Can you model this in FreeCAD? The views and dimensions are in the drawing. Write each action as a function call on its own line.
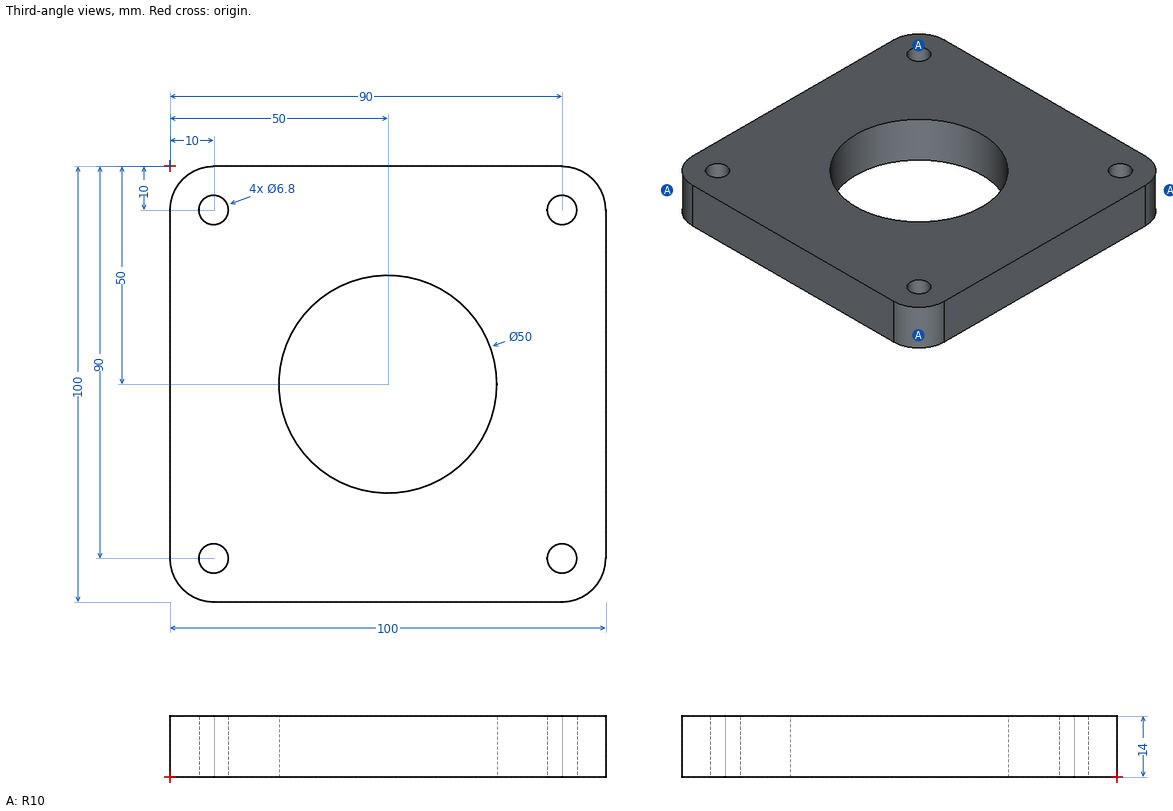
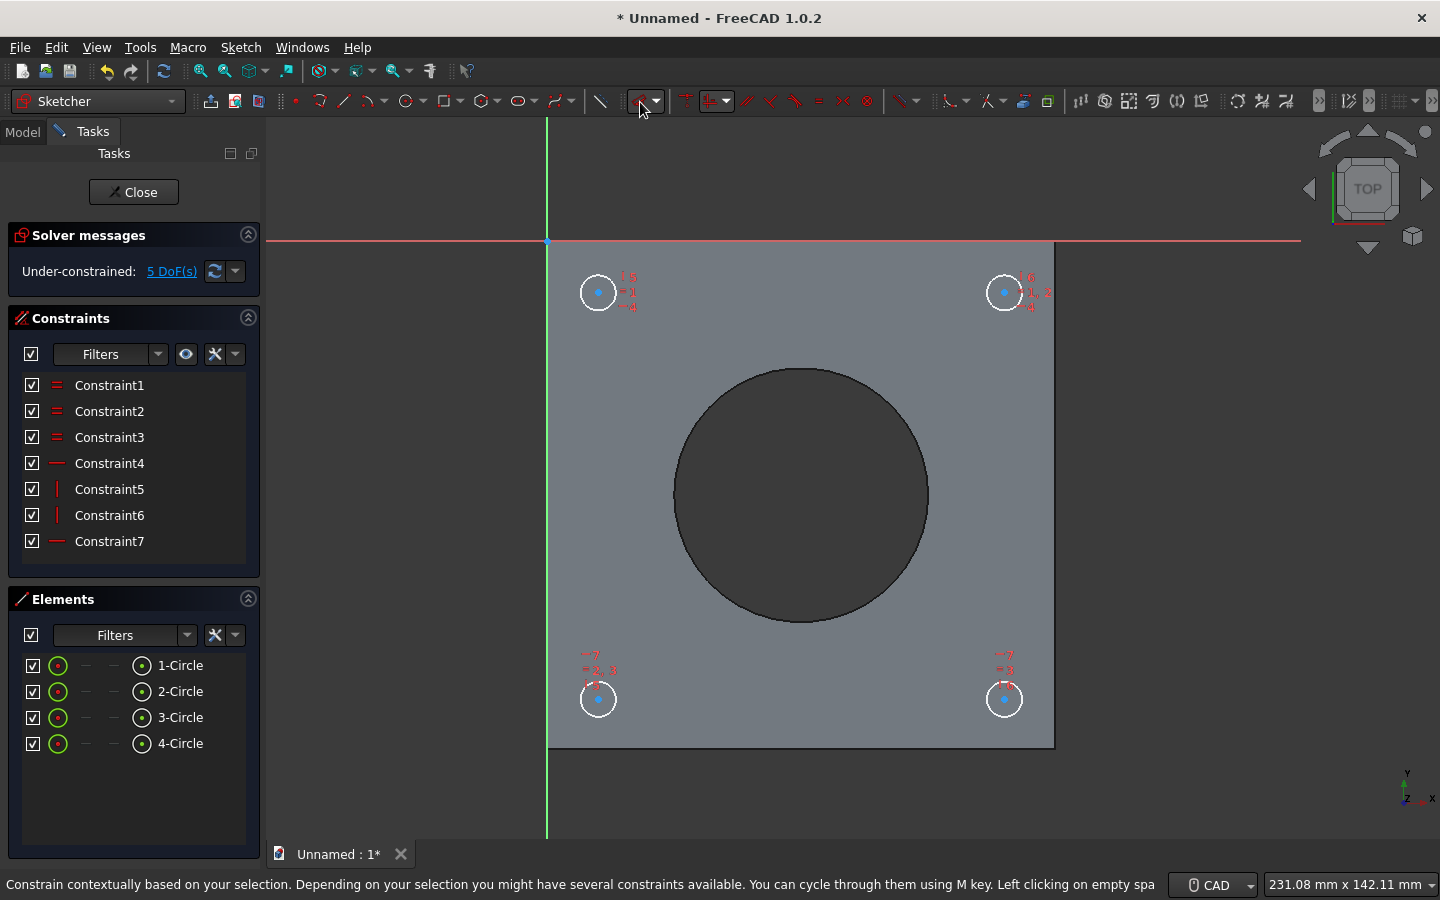
click(611, 280)
click(633, 257)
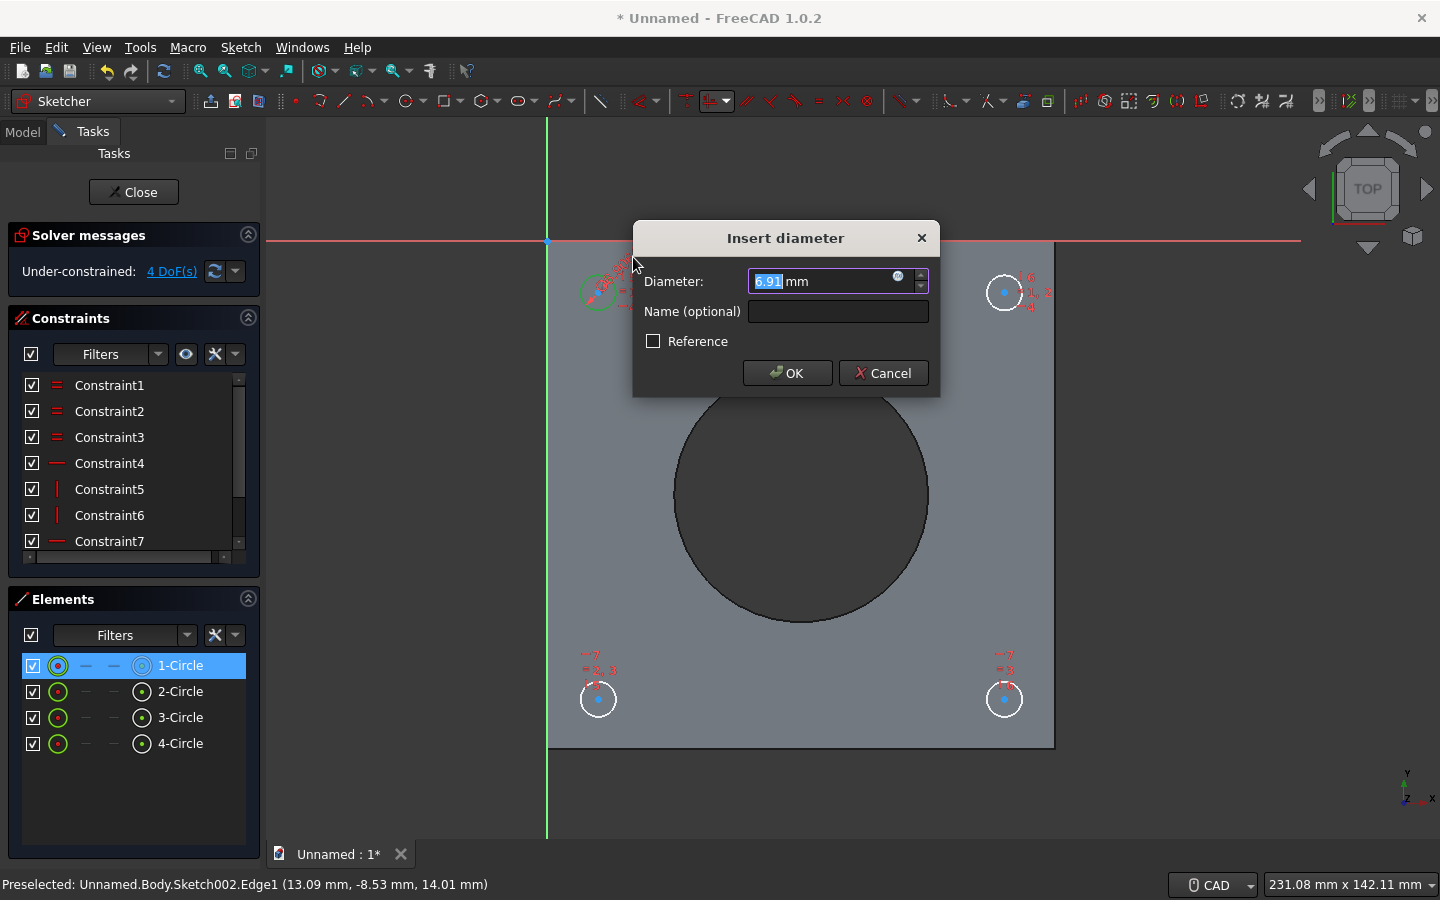
text(6.8)
key(Return)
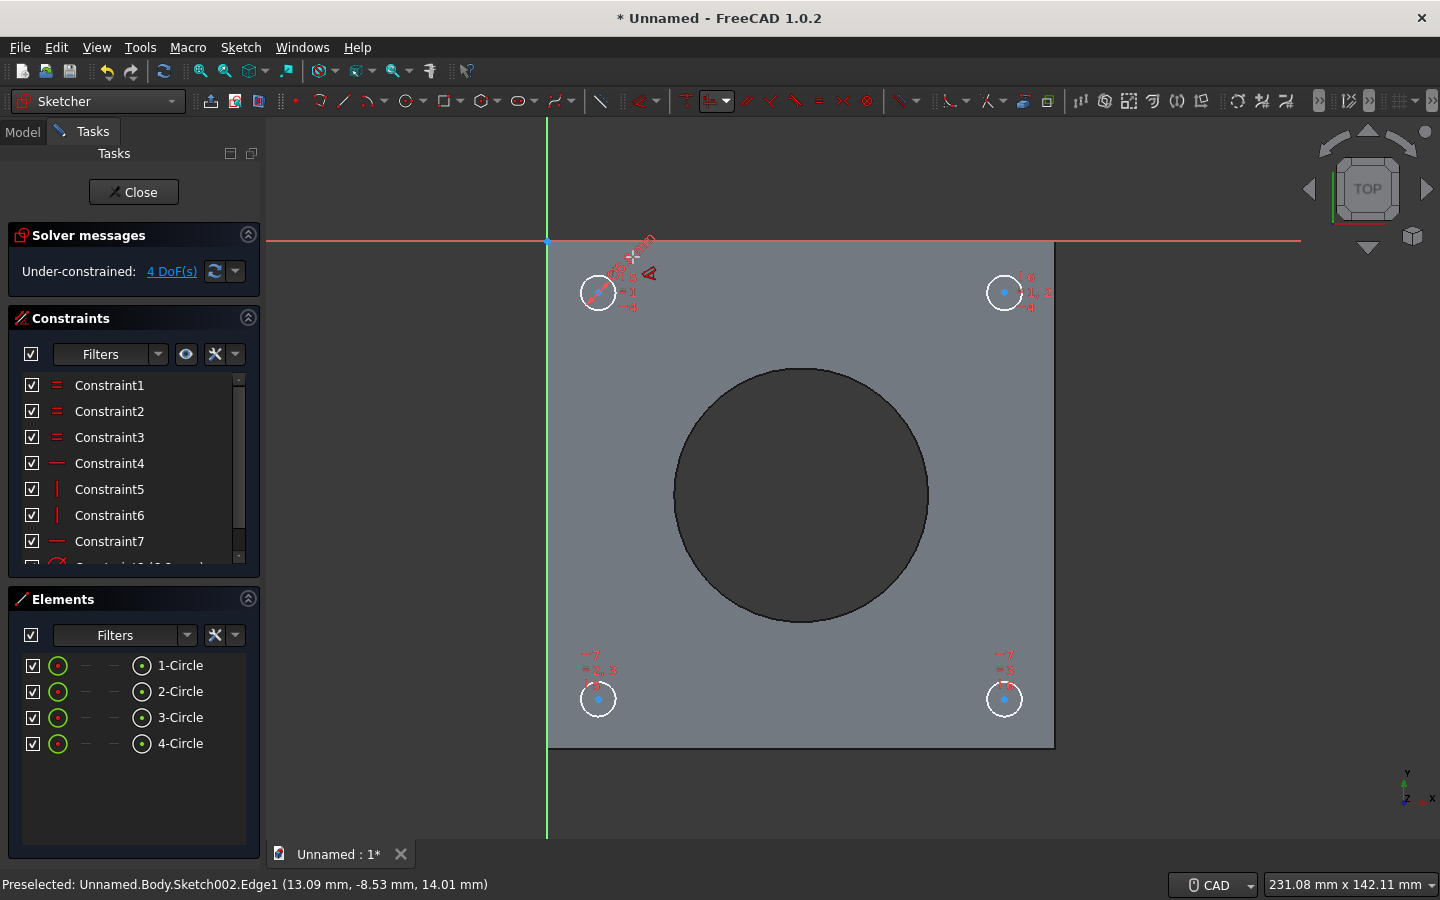
click(598, 293)
click(573, 207)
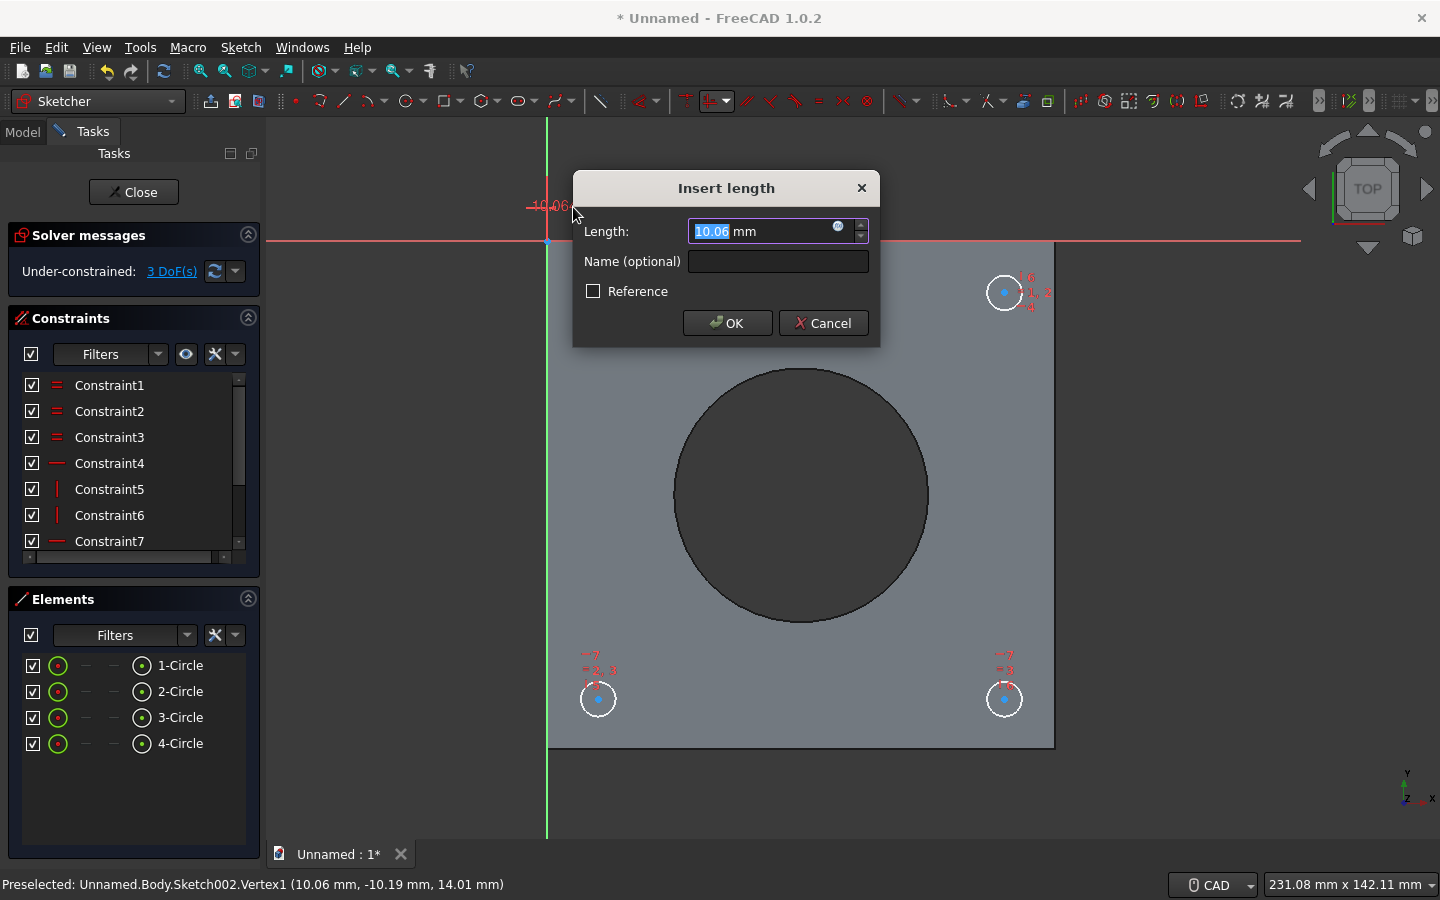
text(10)
key(Return)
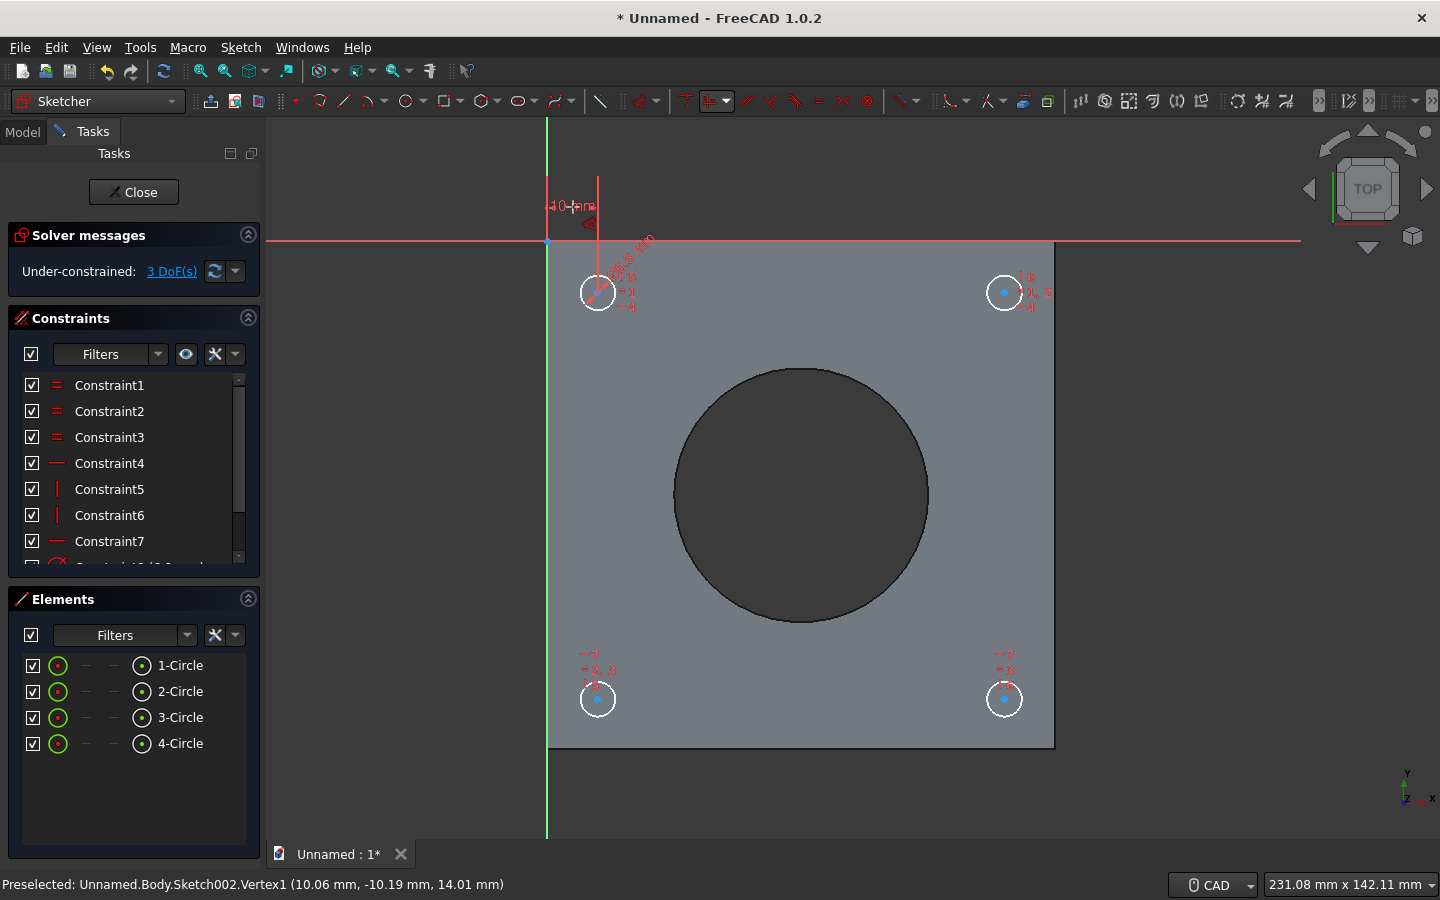
click(598, 293)
click(513, 267)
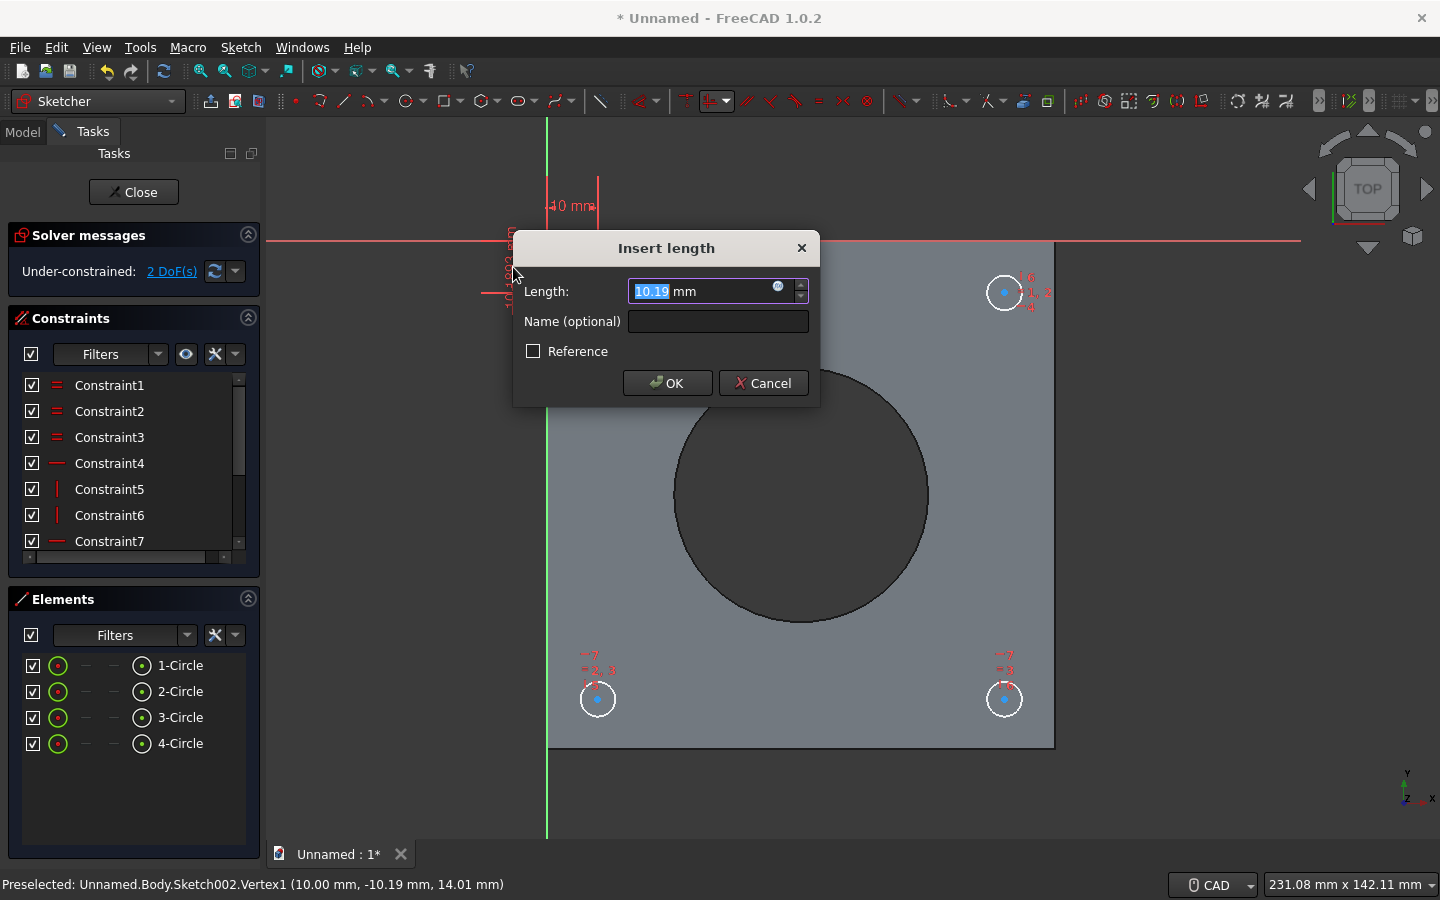
text(10)
key(Return)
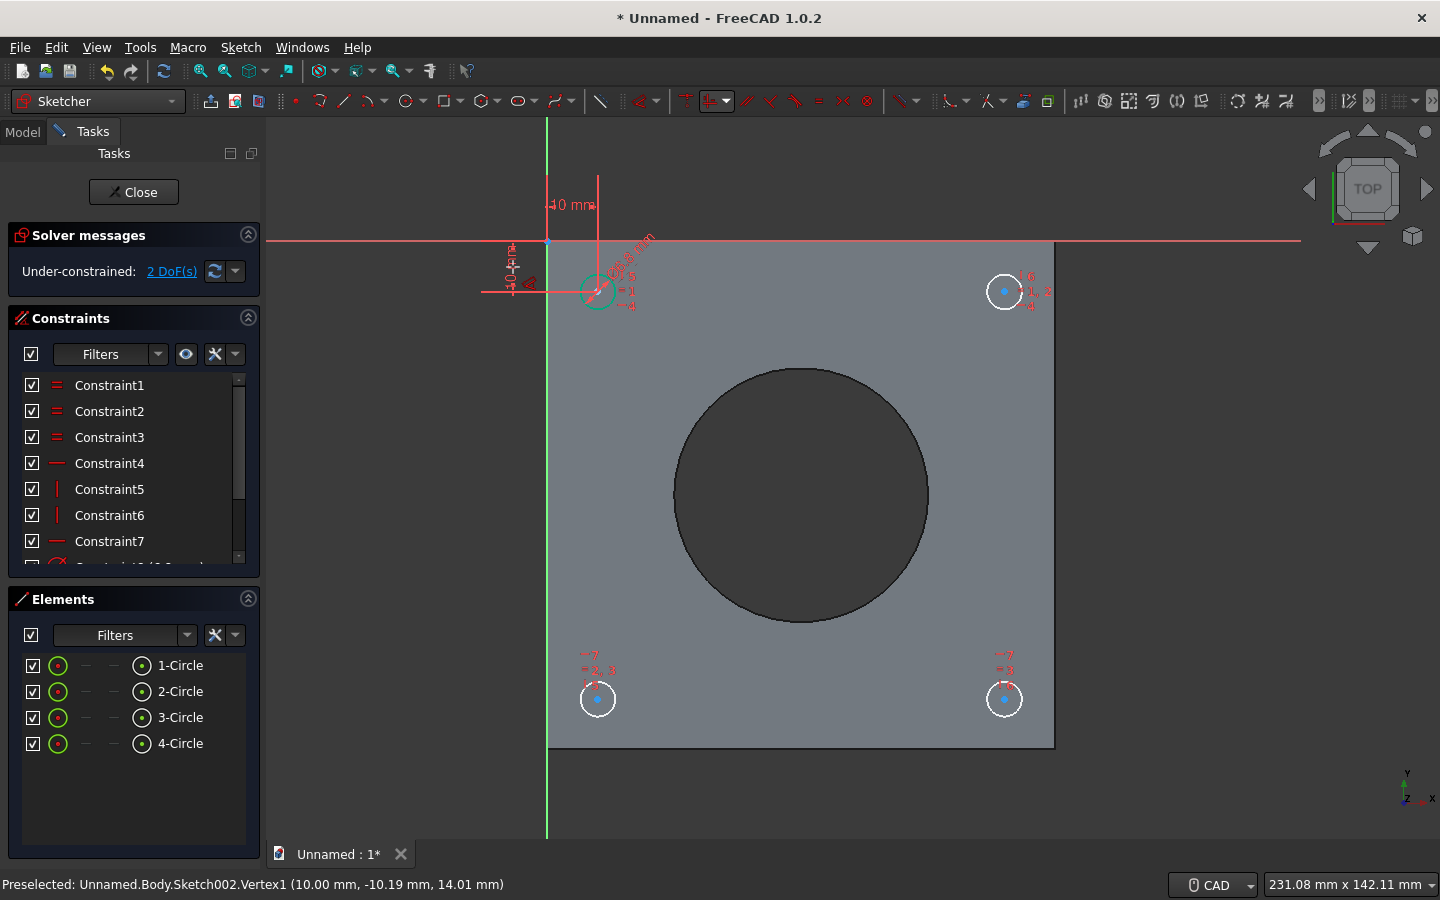
click(1005, 292)
click(776, 207)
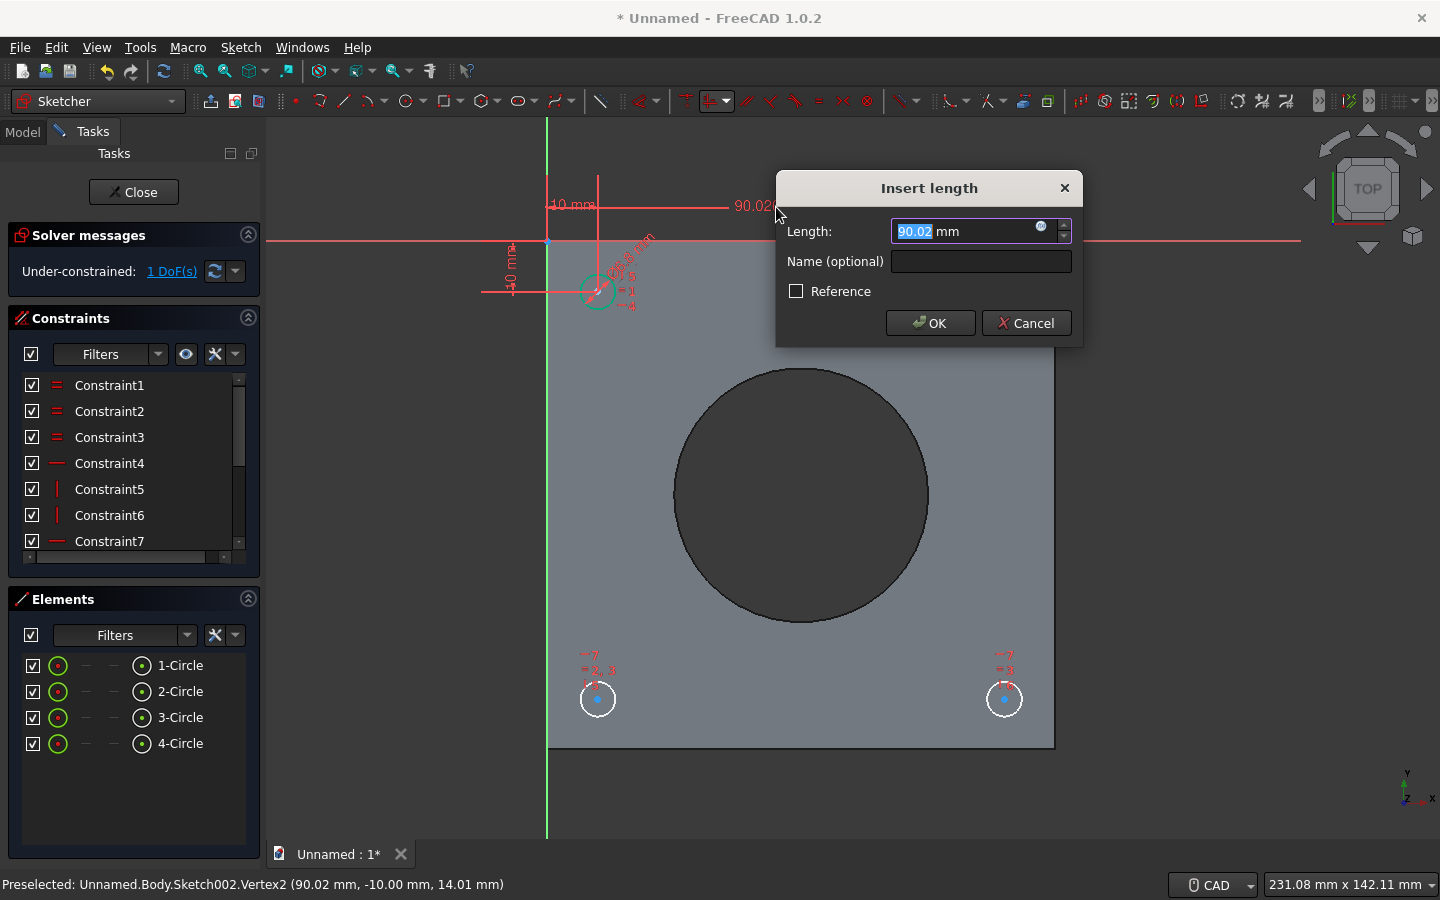
text(90)
key(Return)